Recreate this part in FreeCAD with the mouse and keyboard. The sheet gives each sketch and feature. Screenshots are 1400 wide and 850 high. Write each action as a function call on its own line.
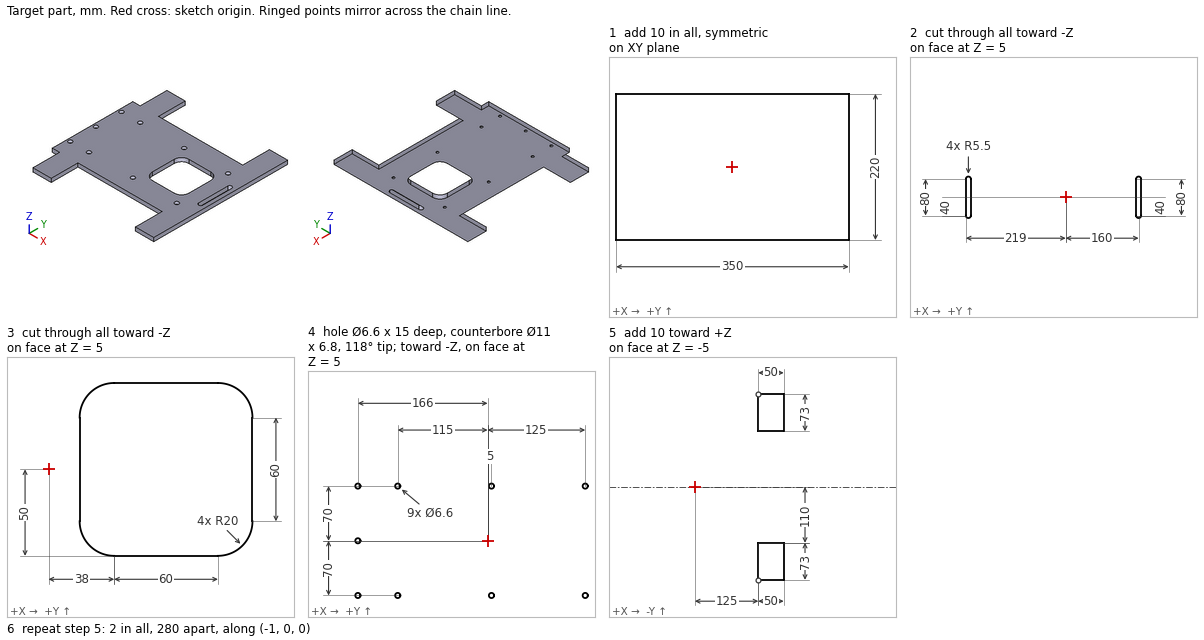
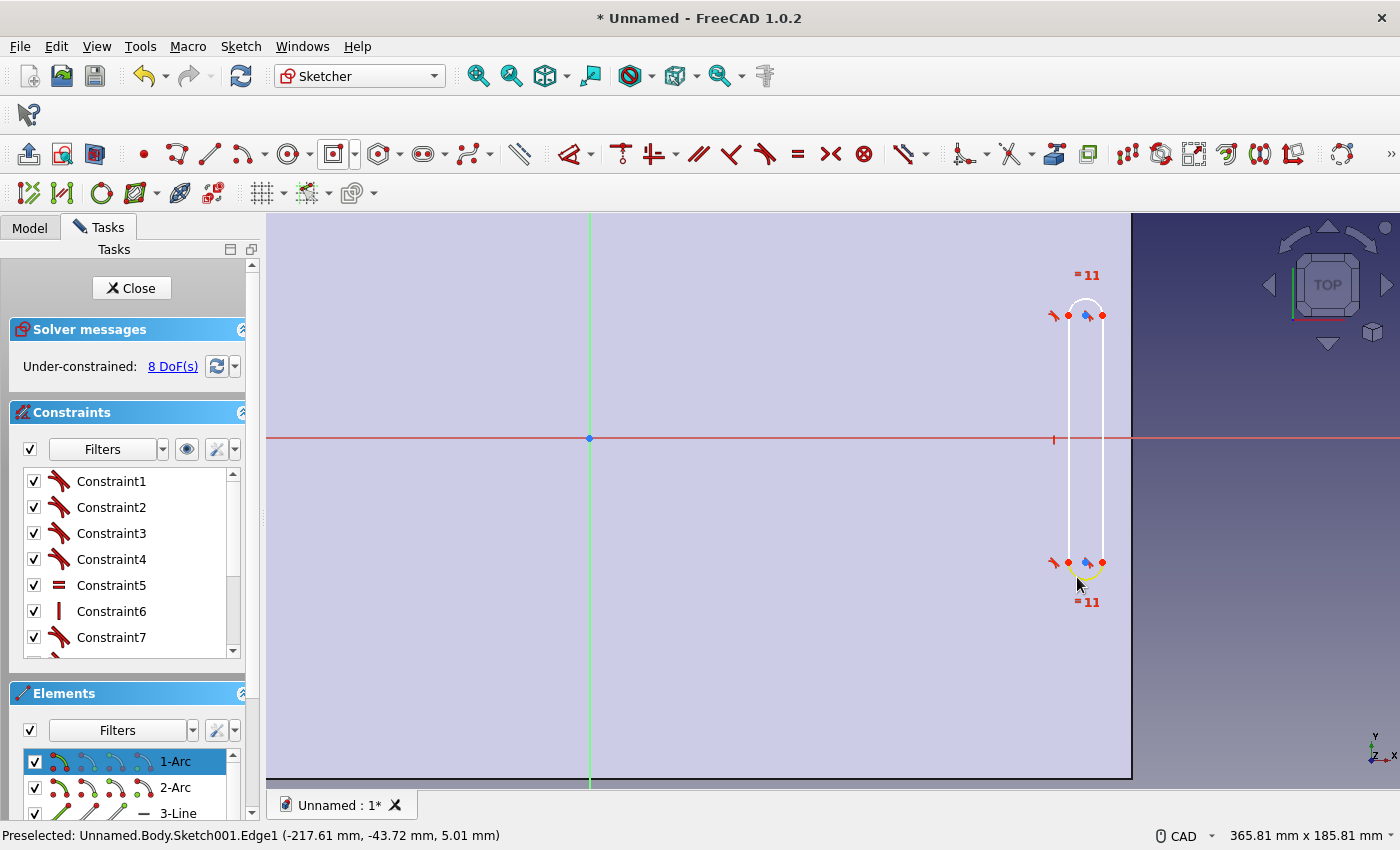
click(1076, 576)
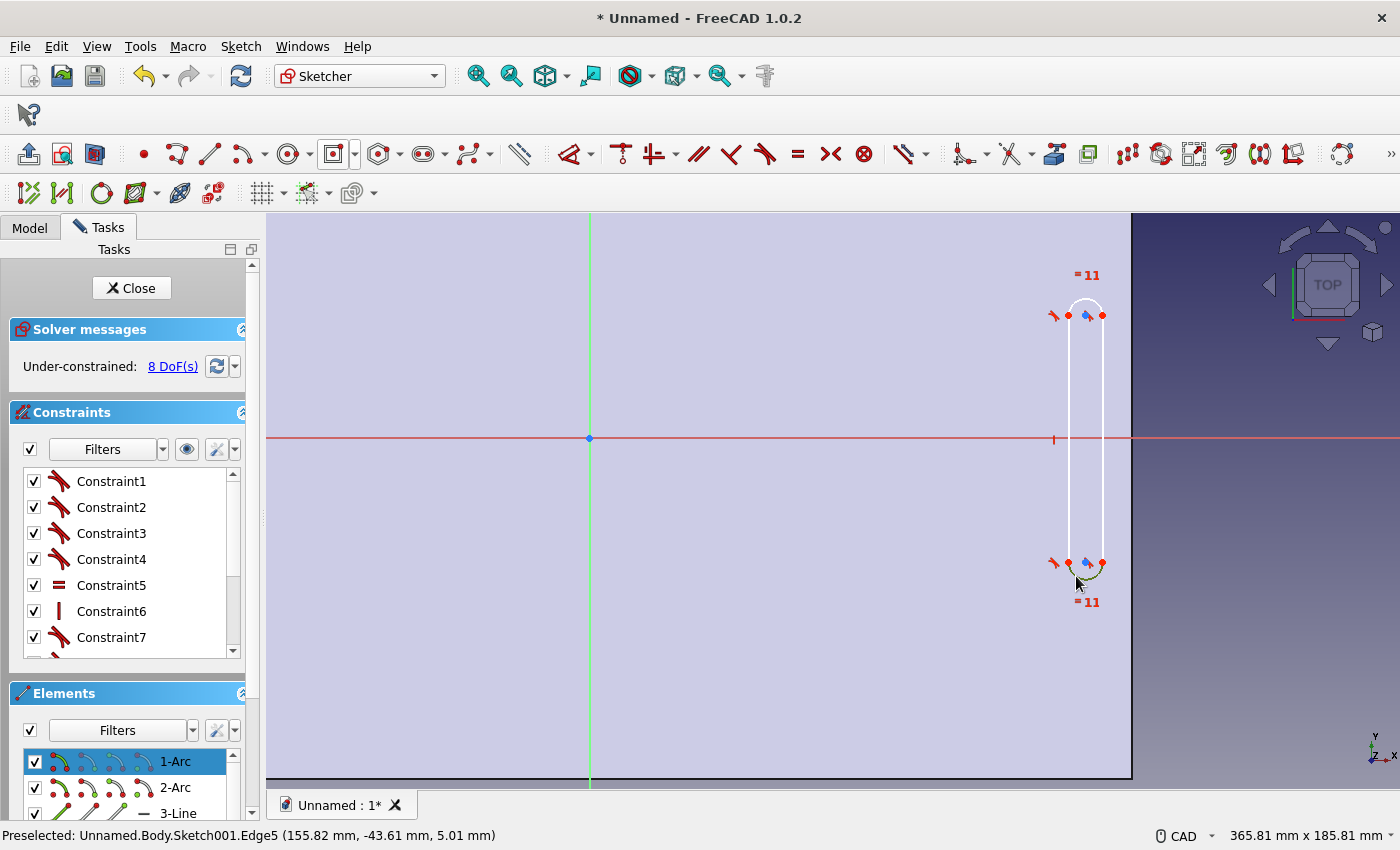
click(798, 154)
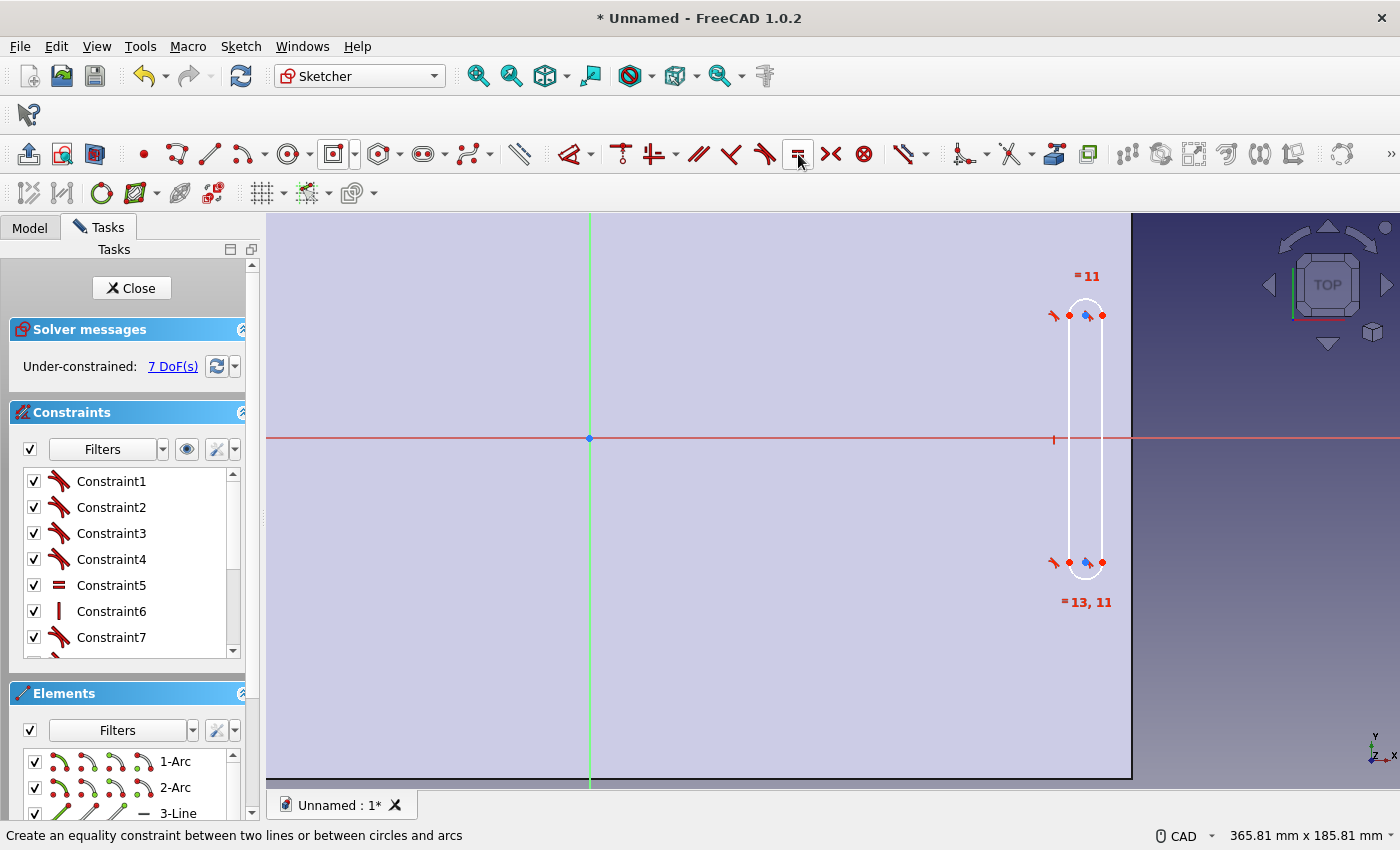
click(568, 154)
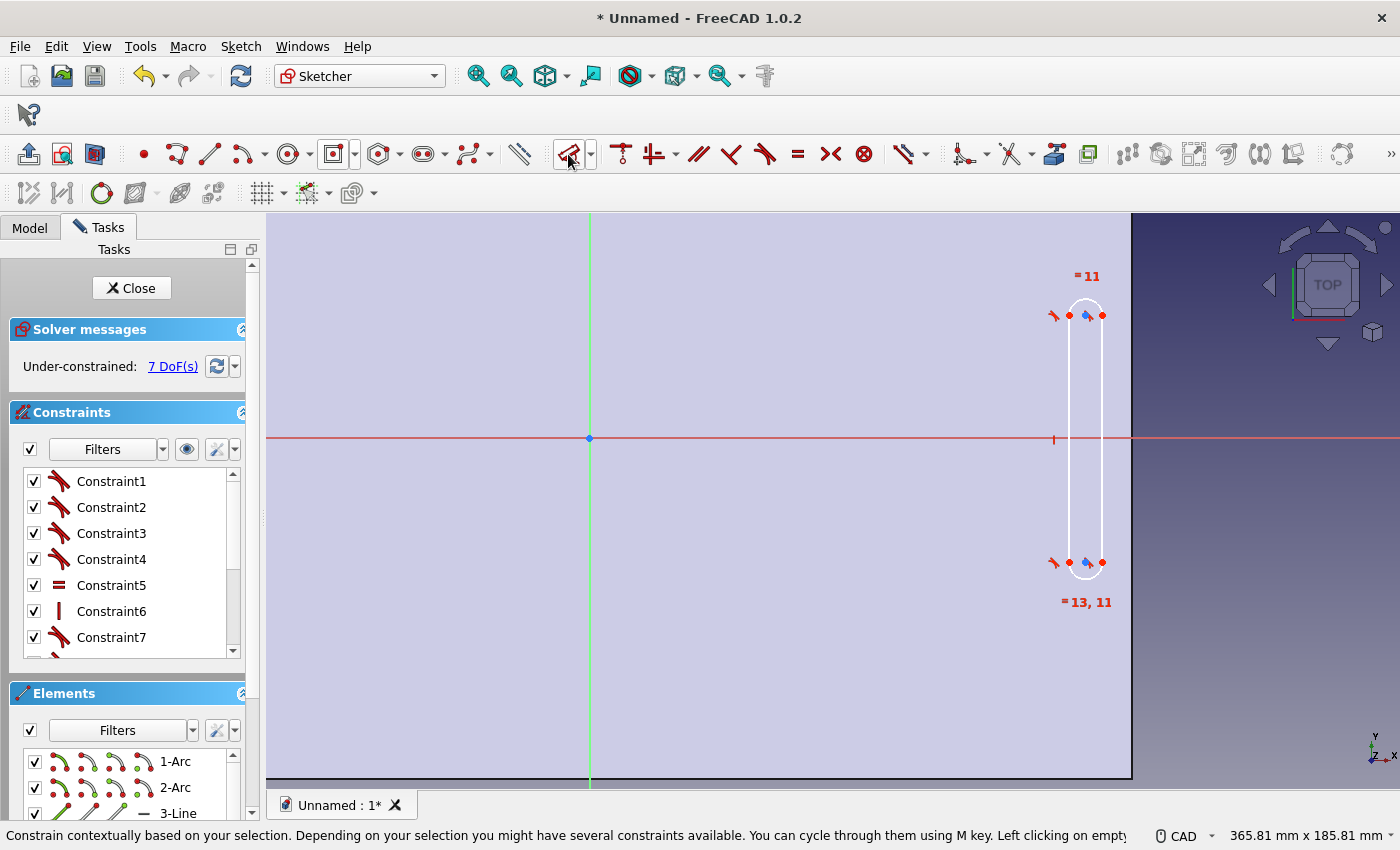
scroll(1078, 577, down, 3)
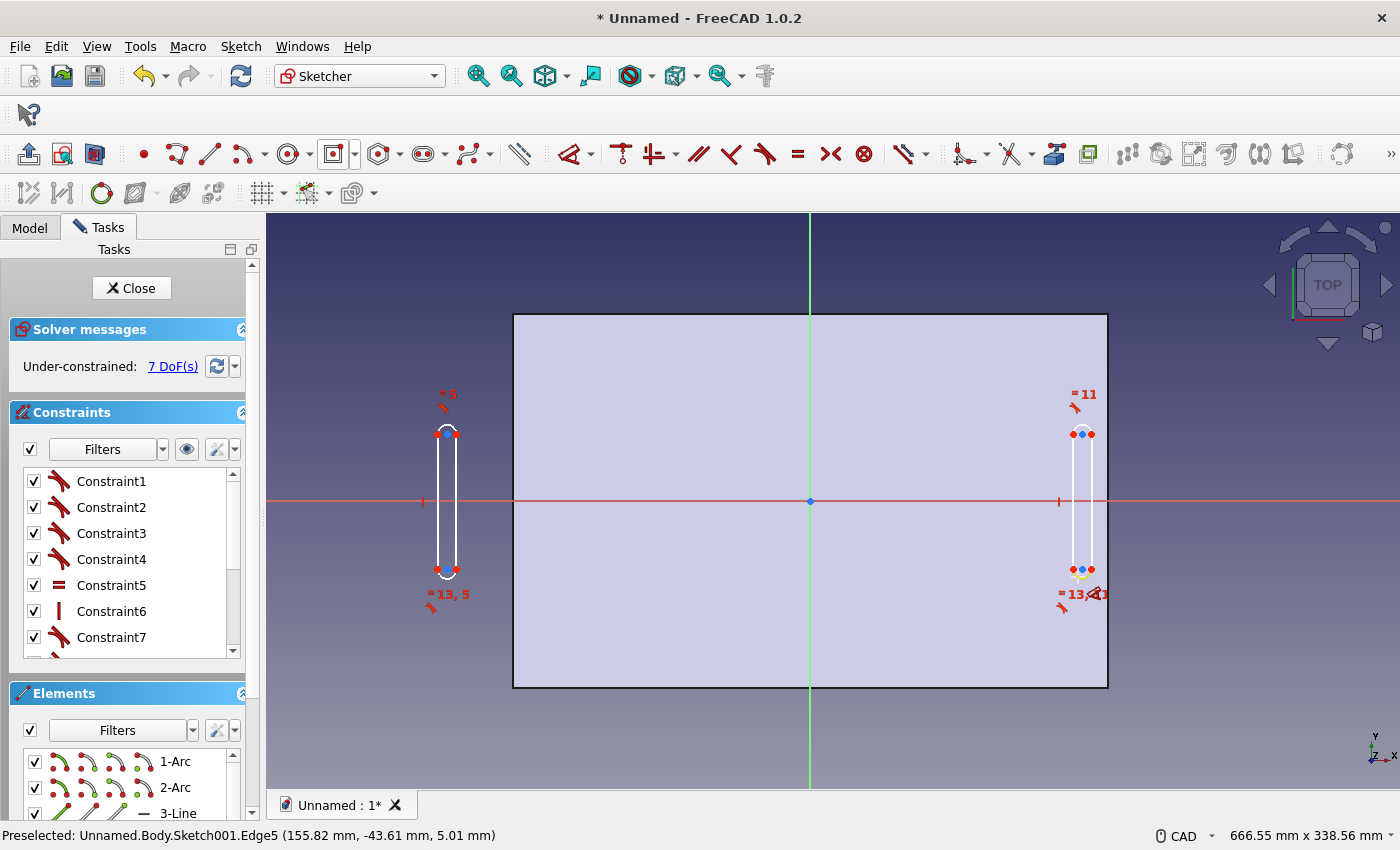
scroll(442, 577, up, 8)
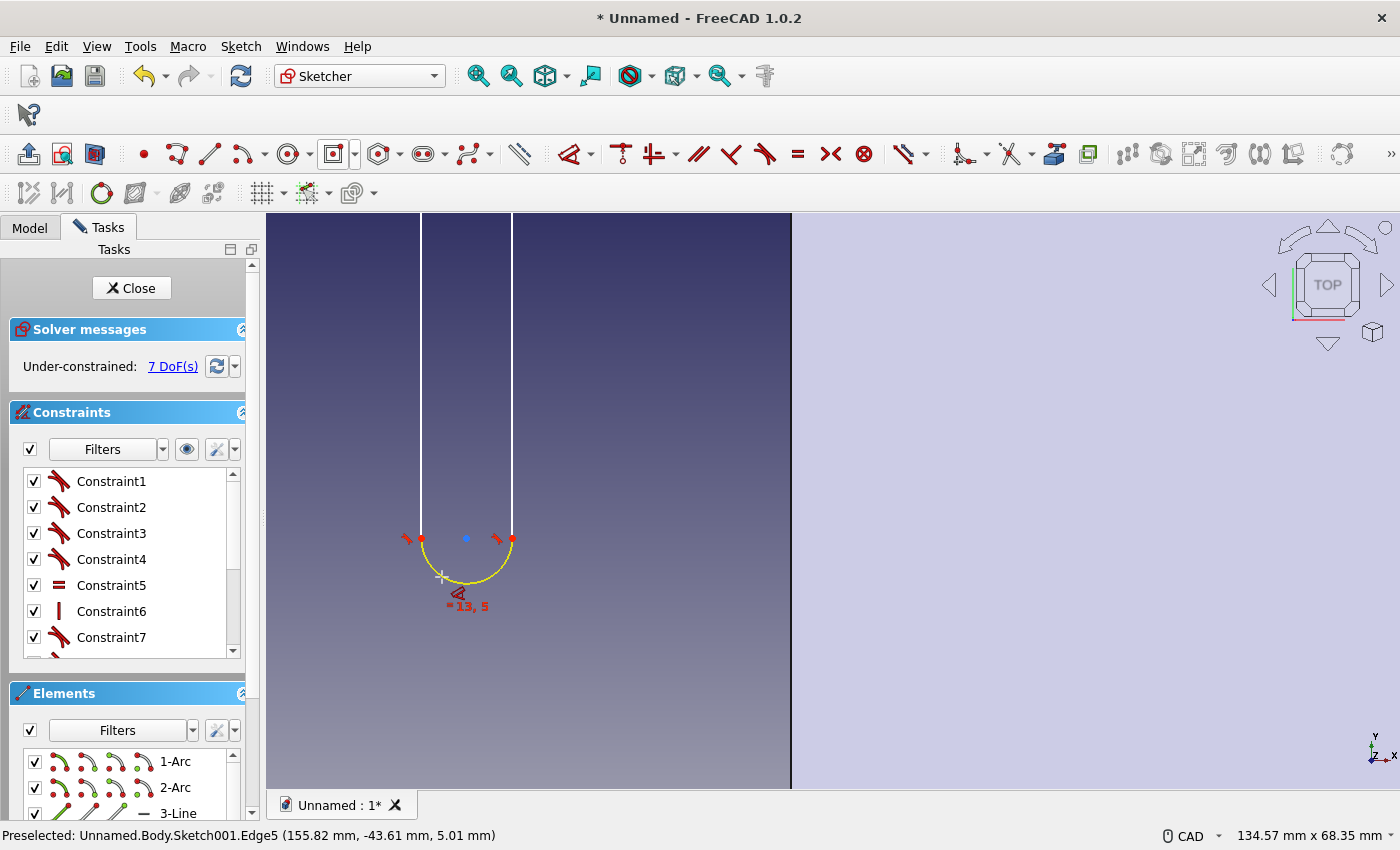
click(440, 575)
click(421, 601)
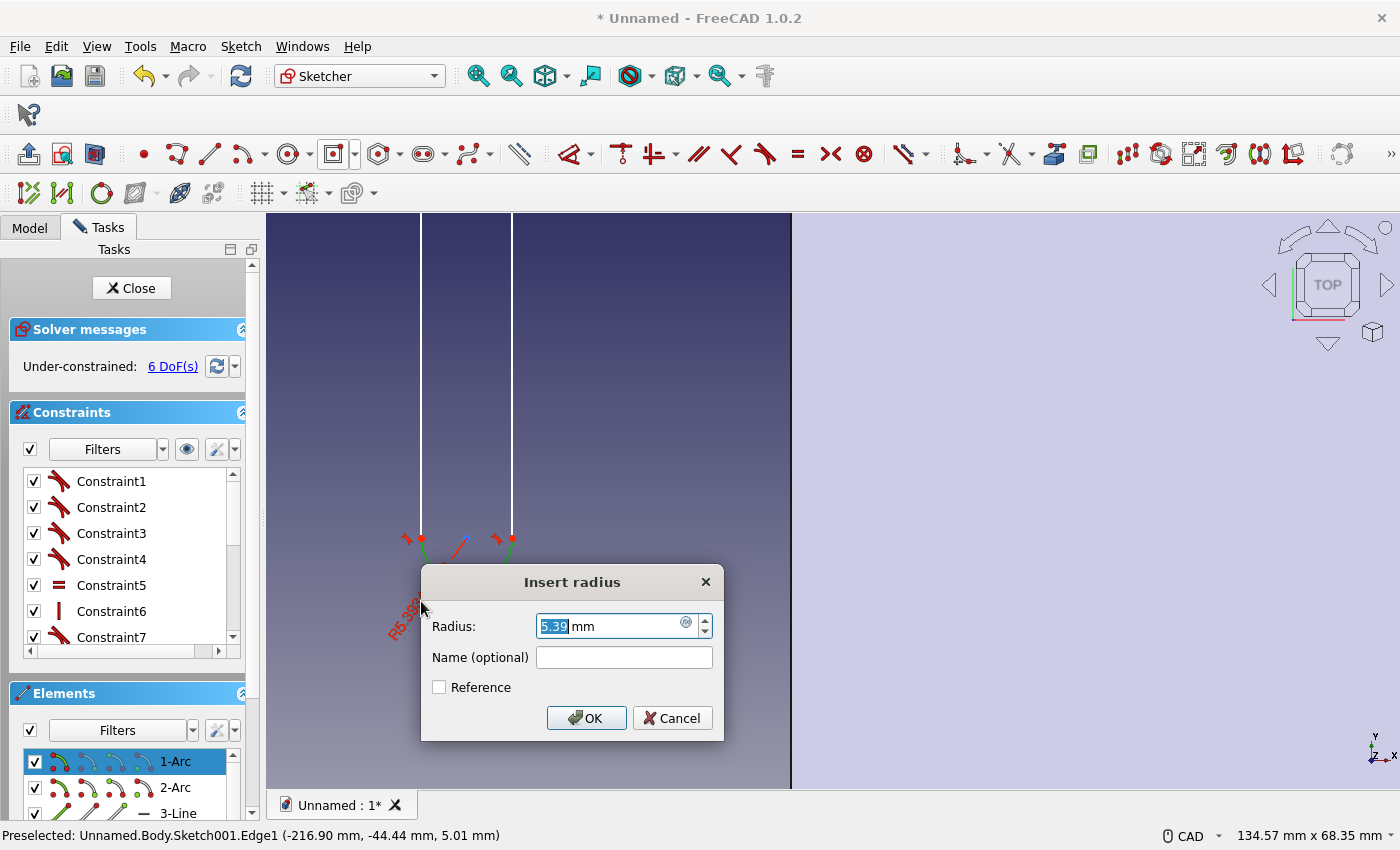
text(5.5)
key(Return)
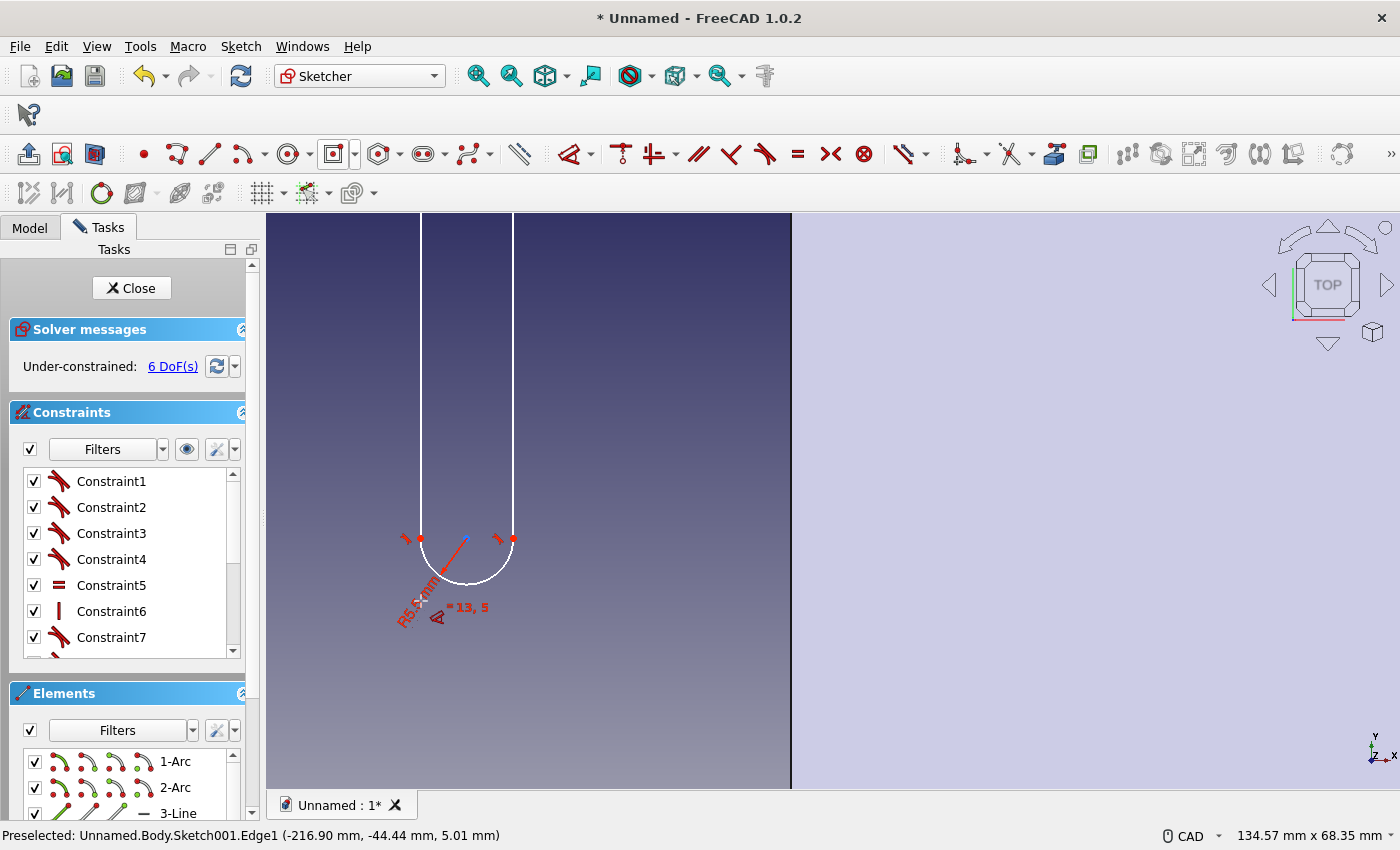
scroll(442, 577, down, 8)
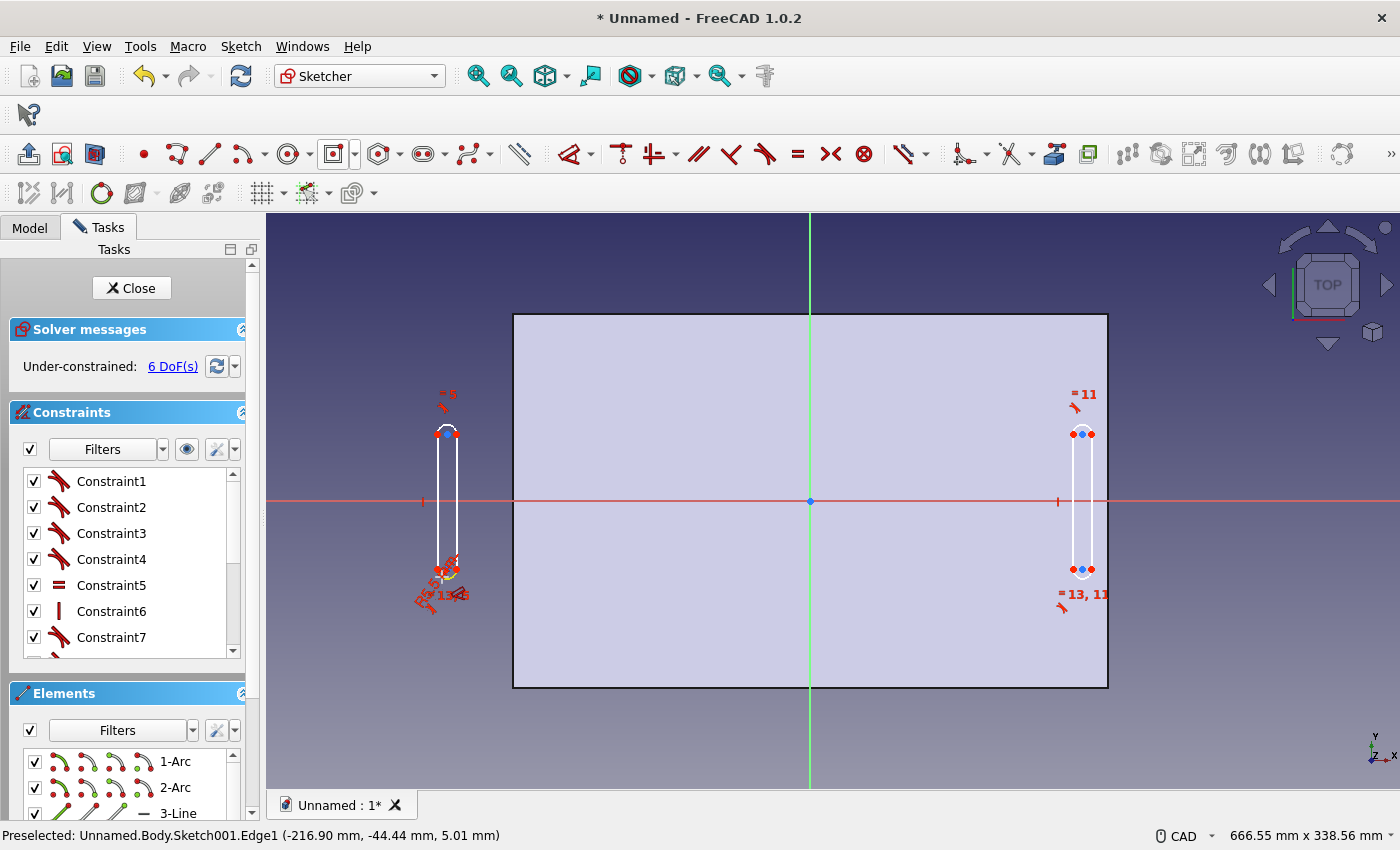
click(438, 529)
click(404, 471)